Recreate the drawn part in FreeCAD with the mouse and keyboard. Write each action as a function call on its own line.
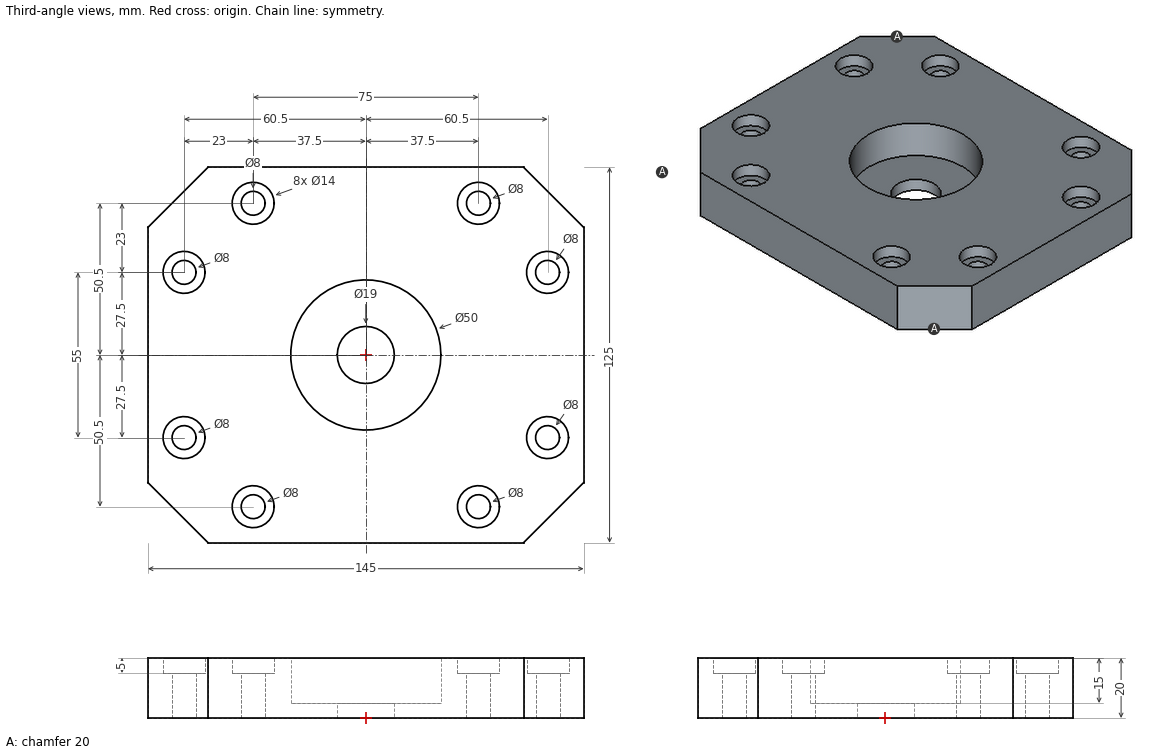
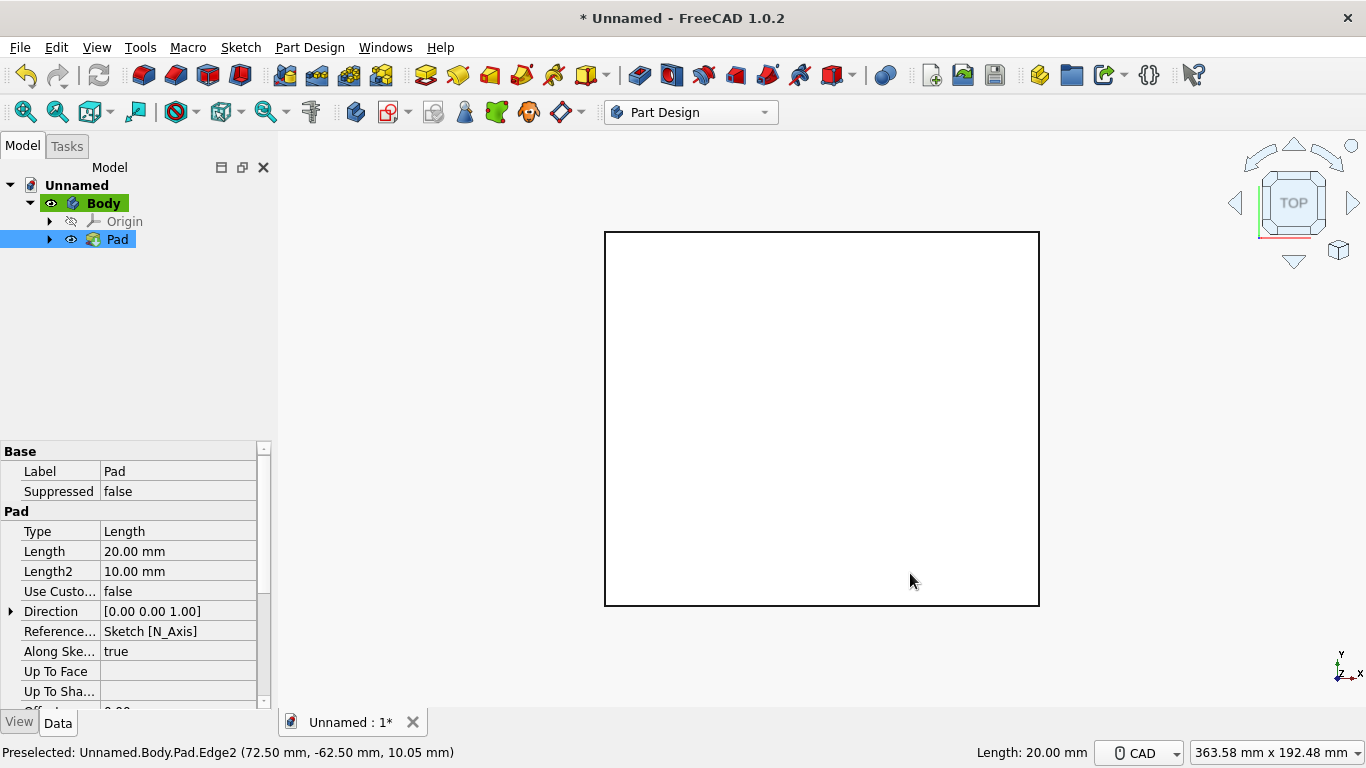
key(1)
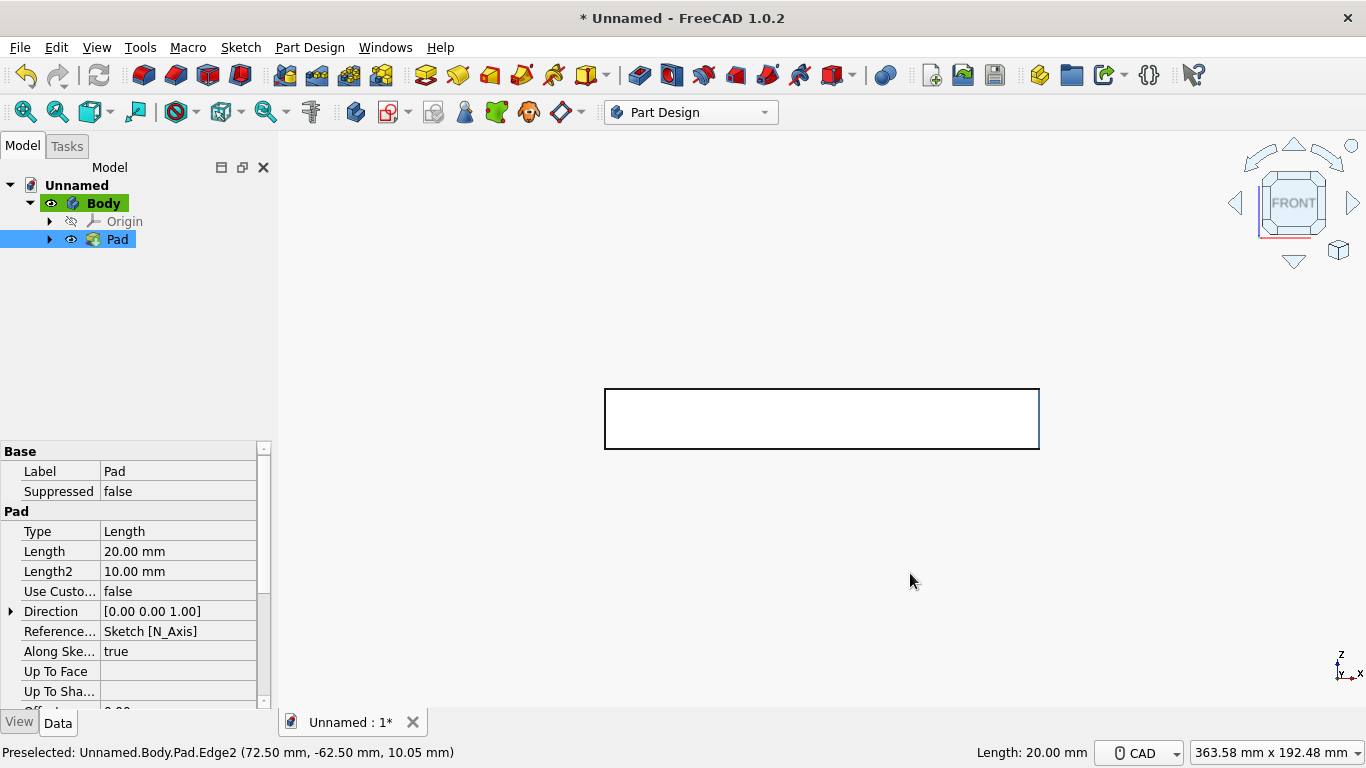
key(v)
key(f)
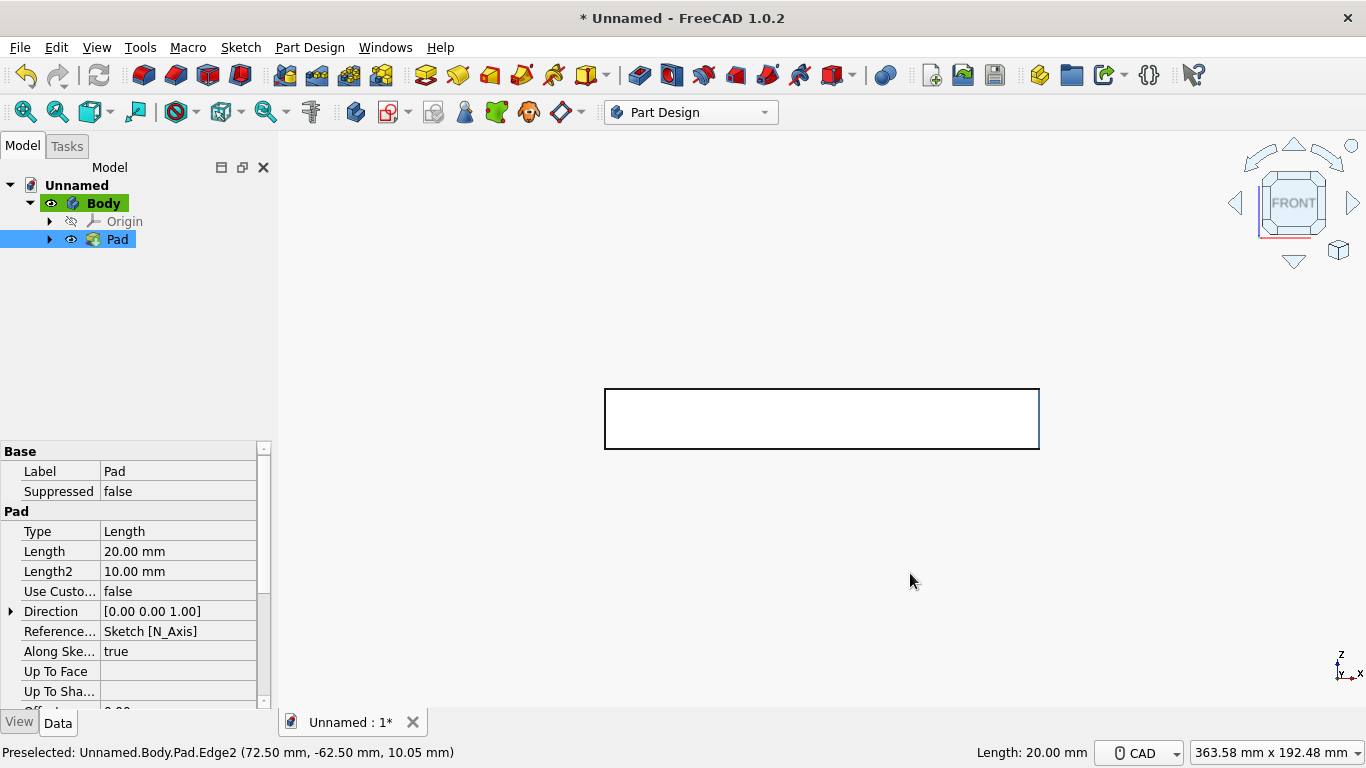
click(605, 418, ctrl)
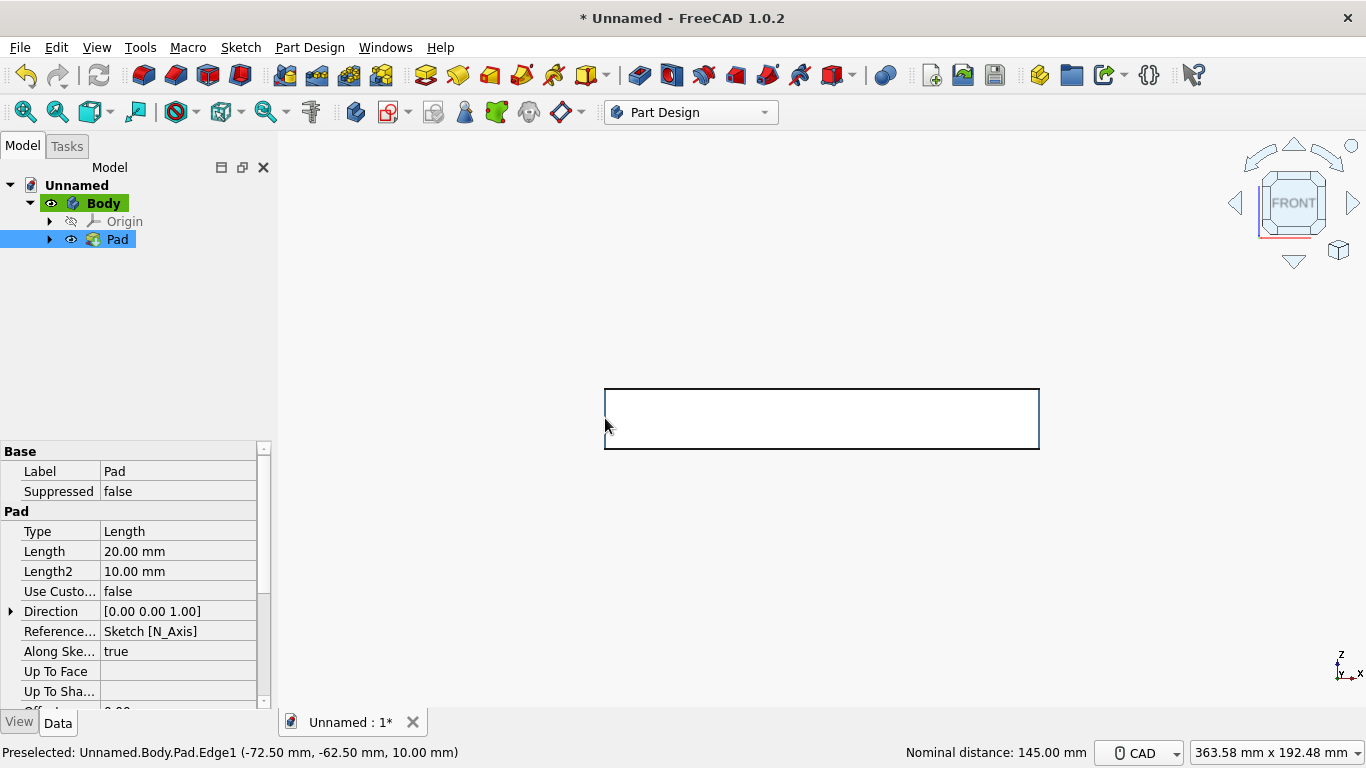
key(3)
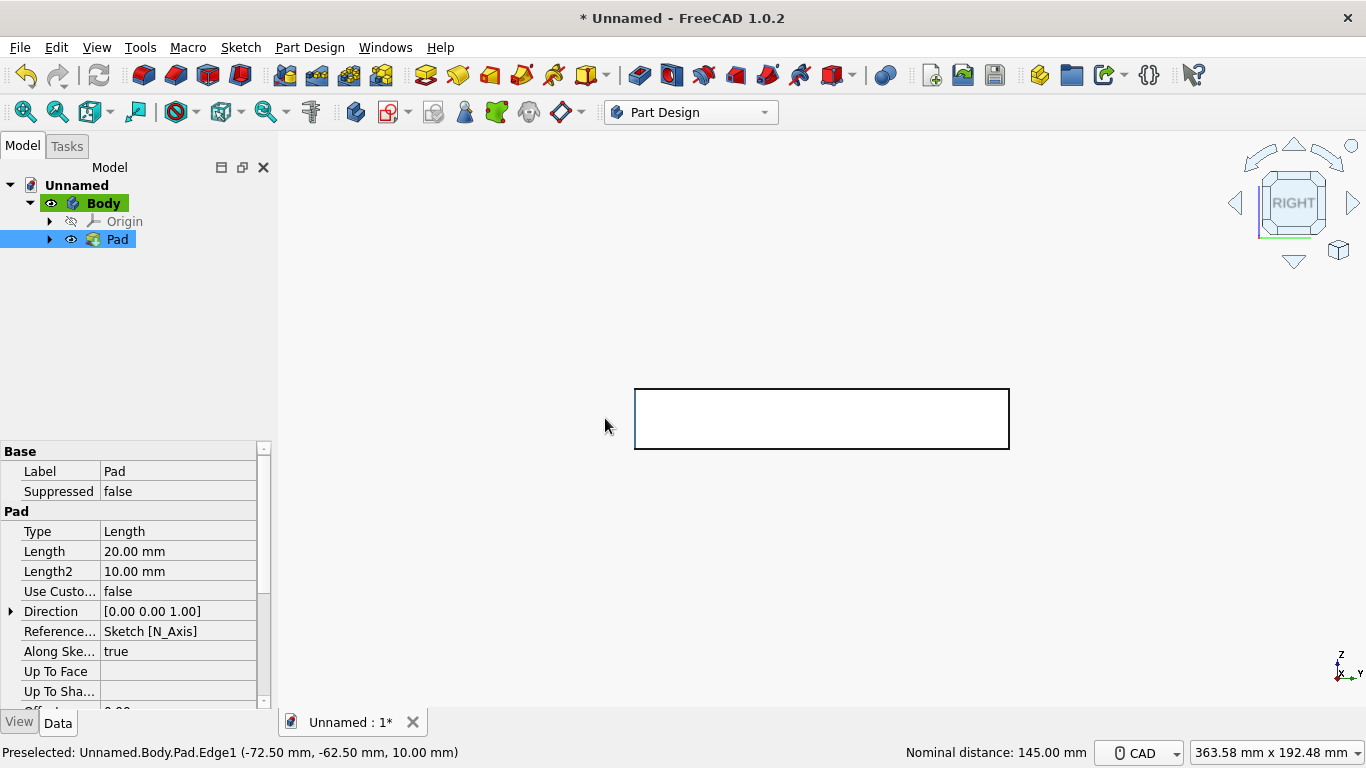
key(v)
key(f)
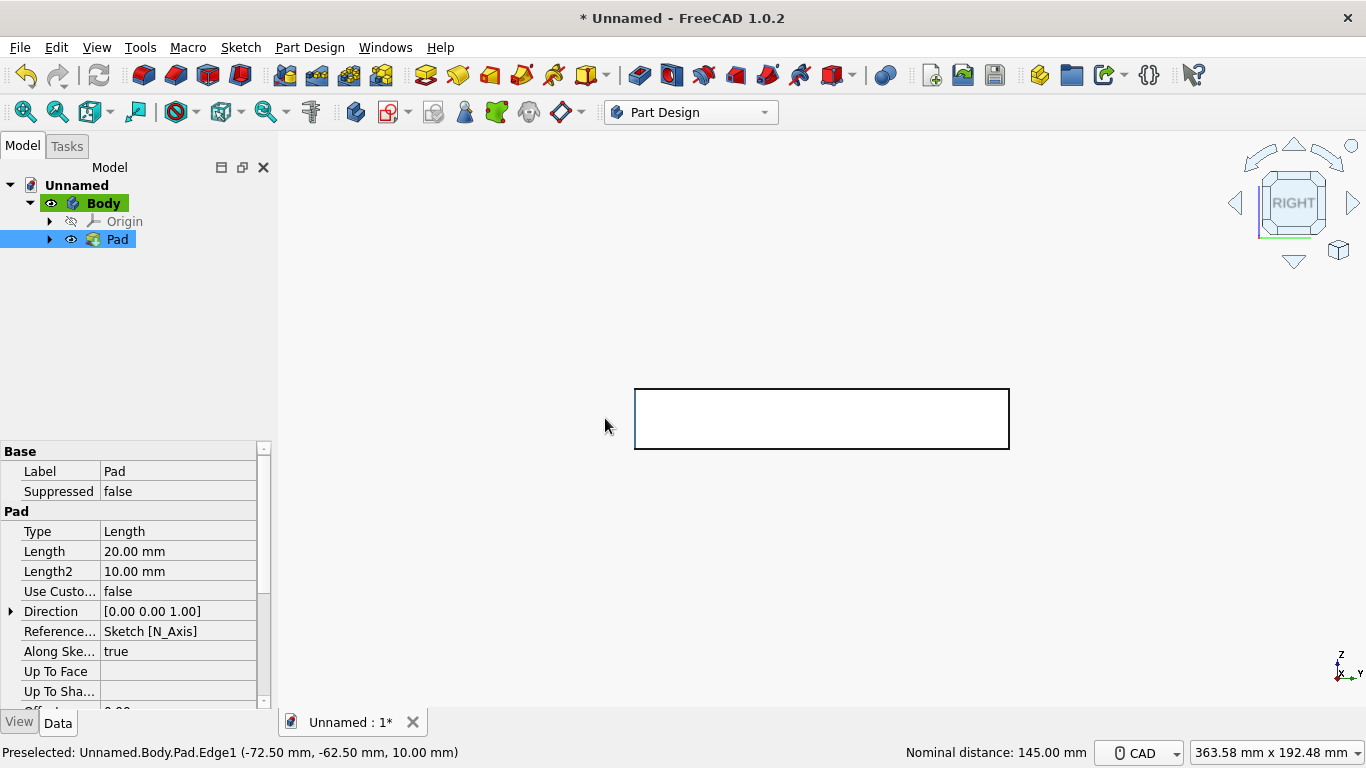
click(1009, 418, ctrl)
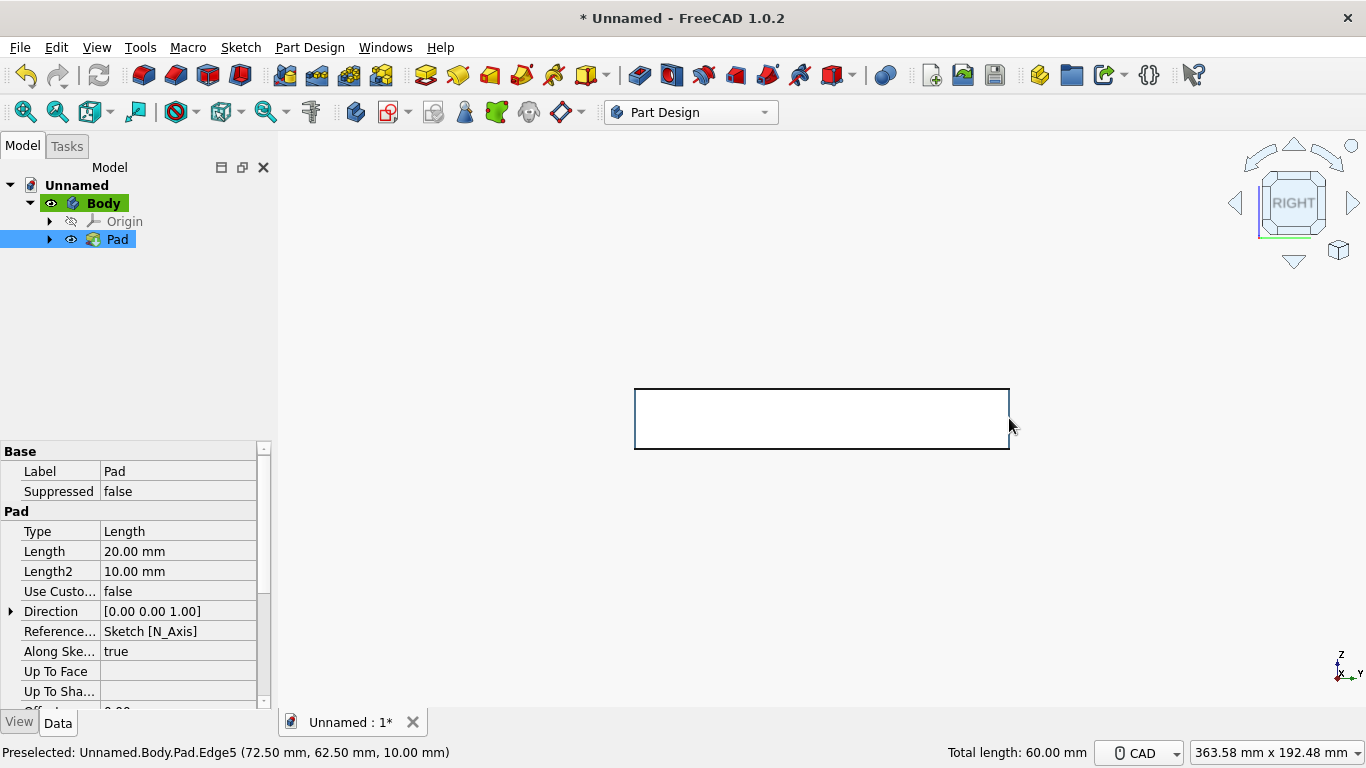
key(5)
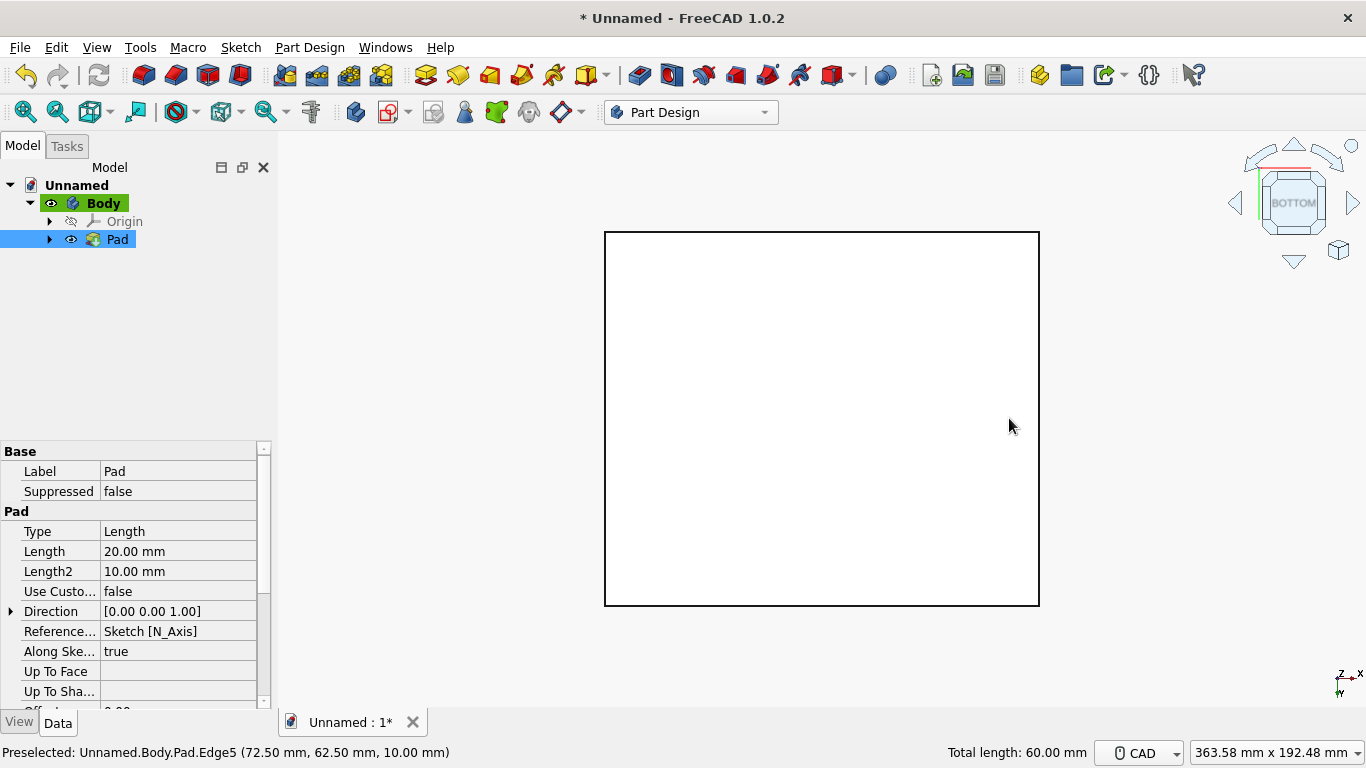
key(4)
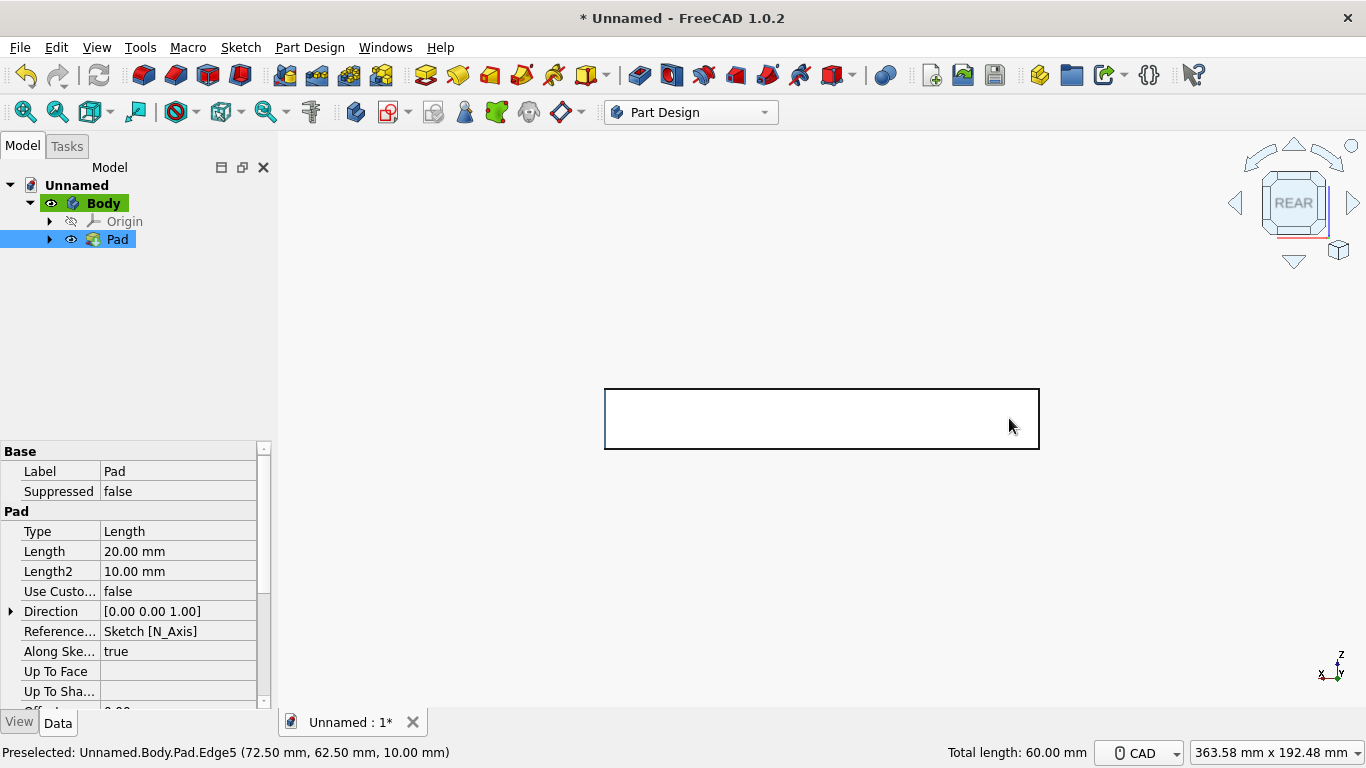
click(26, 112)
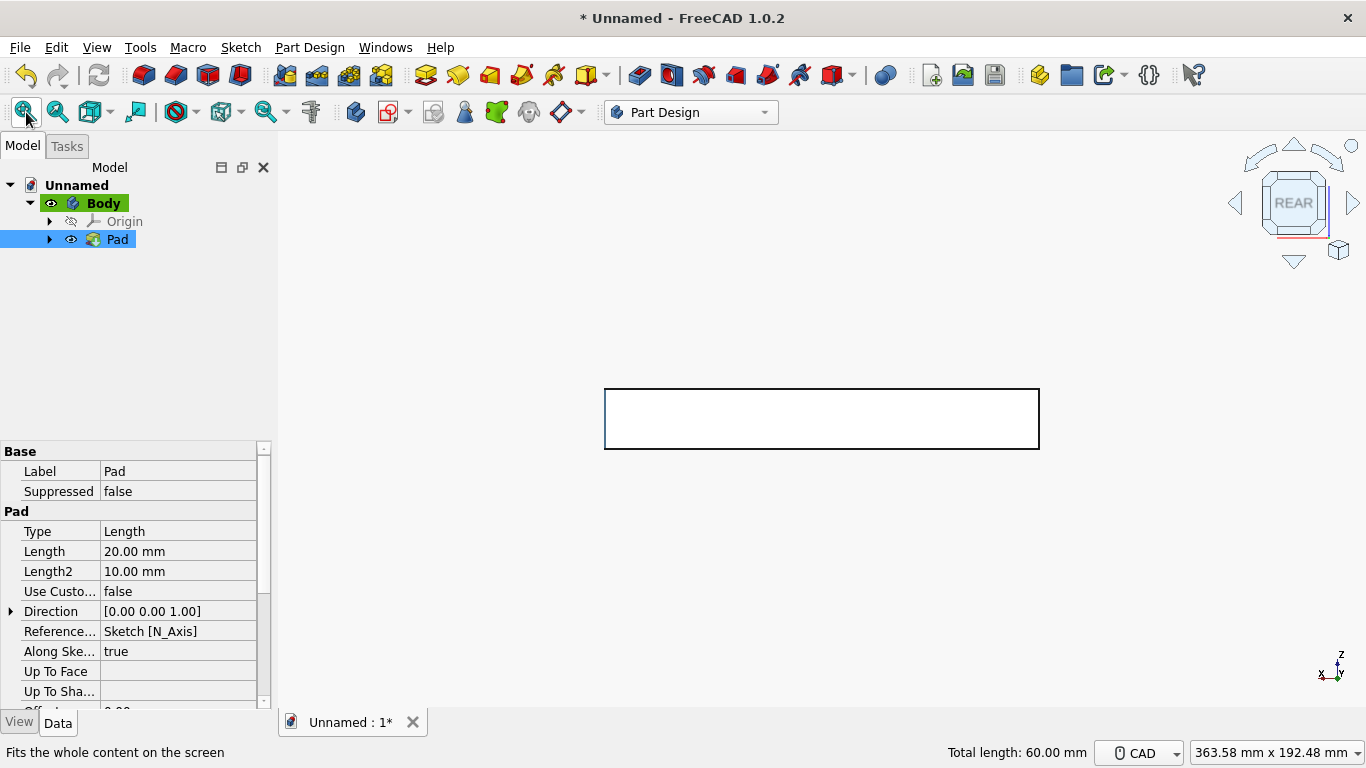
click(1039, 418, ctrl)